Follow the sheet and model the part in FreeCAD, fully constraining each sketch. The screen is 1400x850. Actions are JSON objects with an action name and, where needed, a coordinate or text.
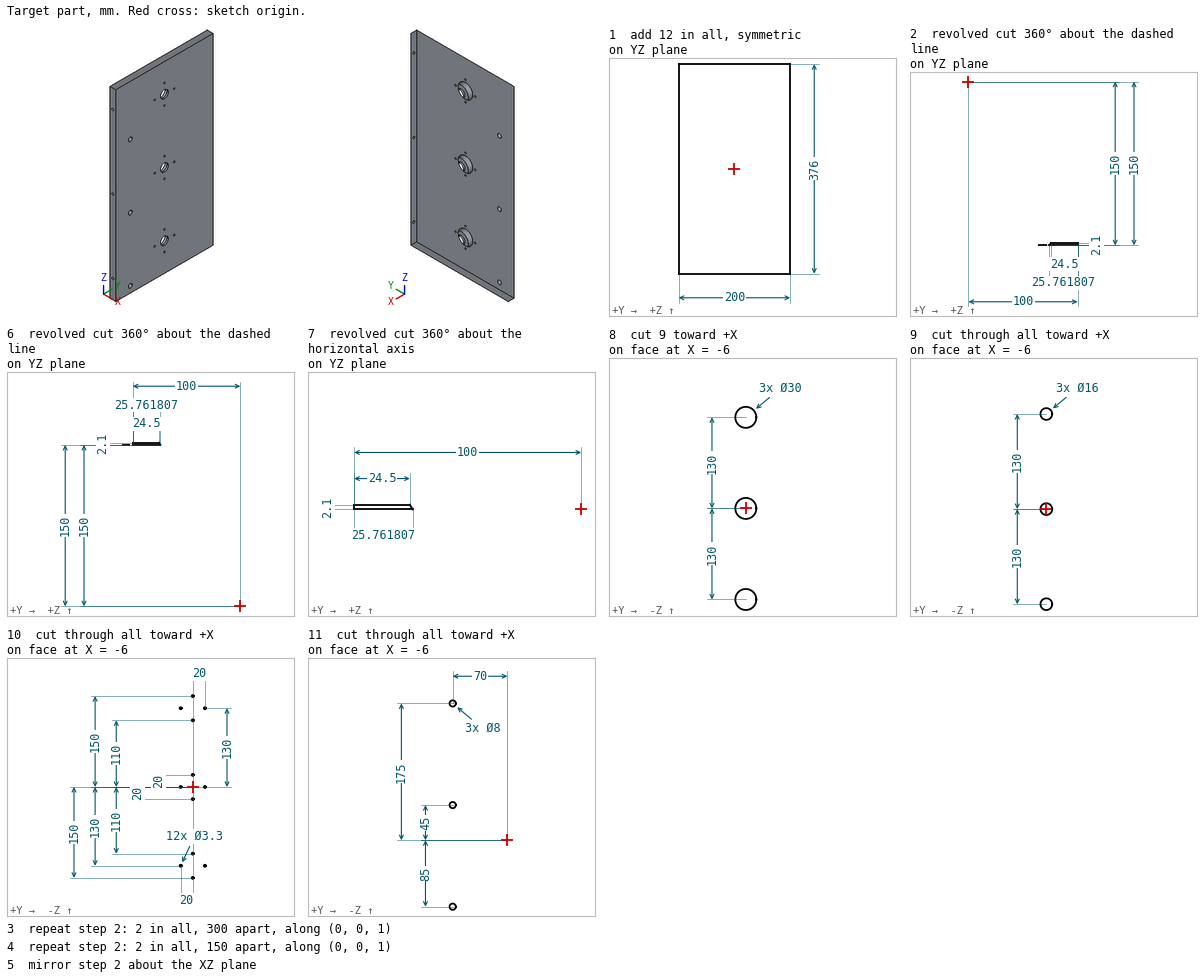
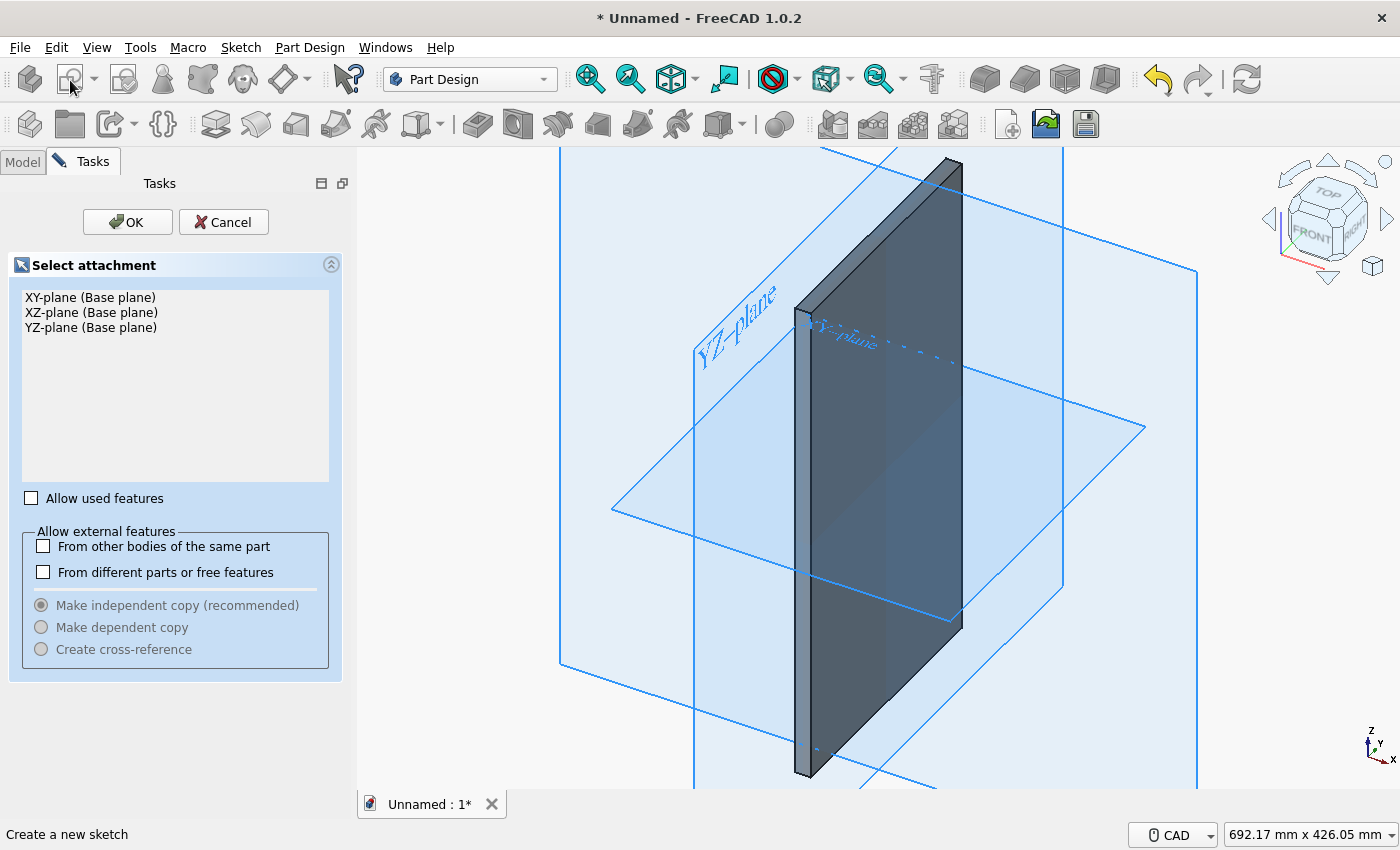
{"action": "left_click", "coordinate": [82, 328]}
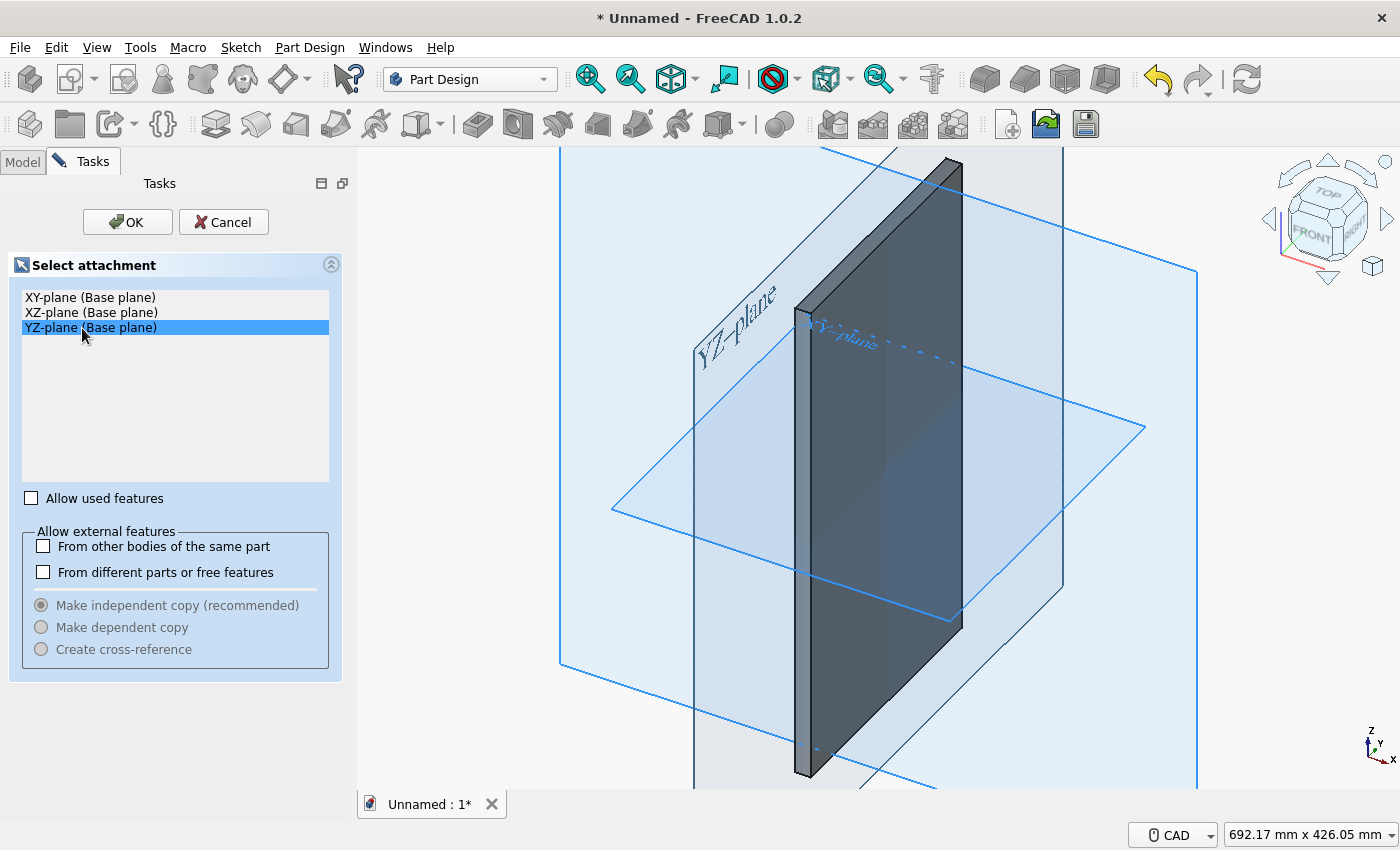
{"action": "left_click", "coordinate": [128, 222]}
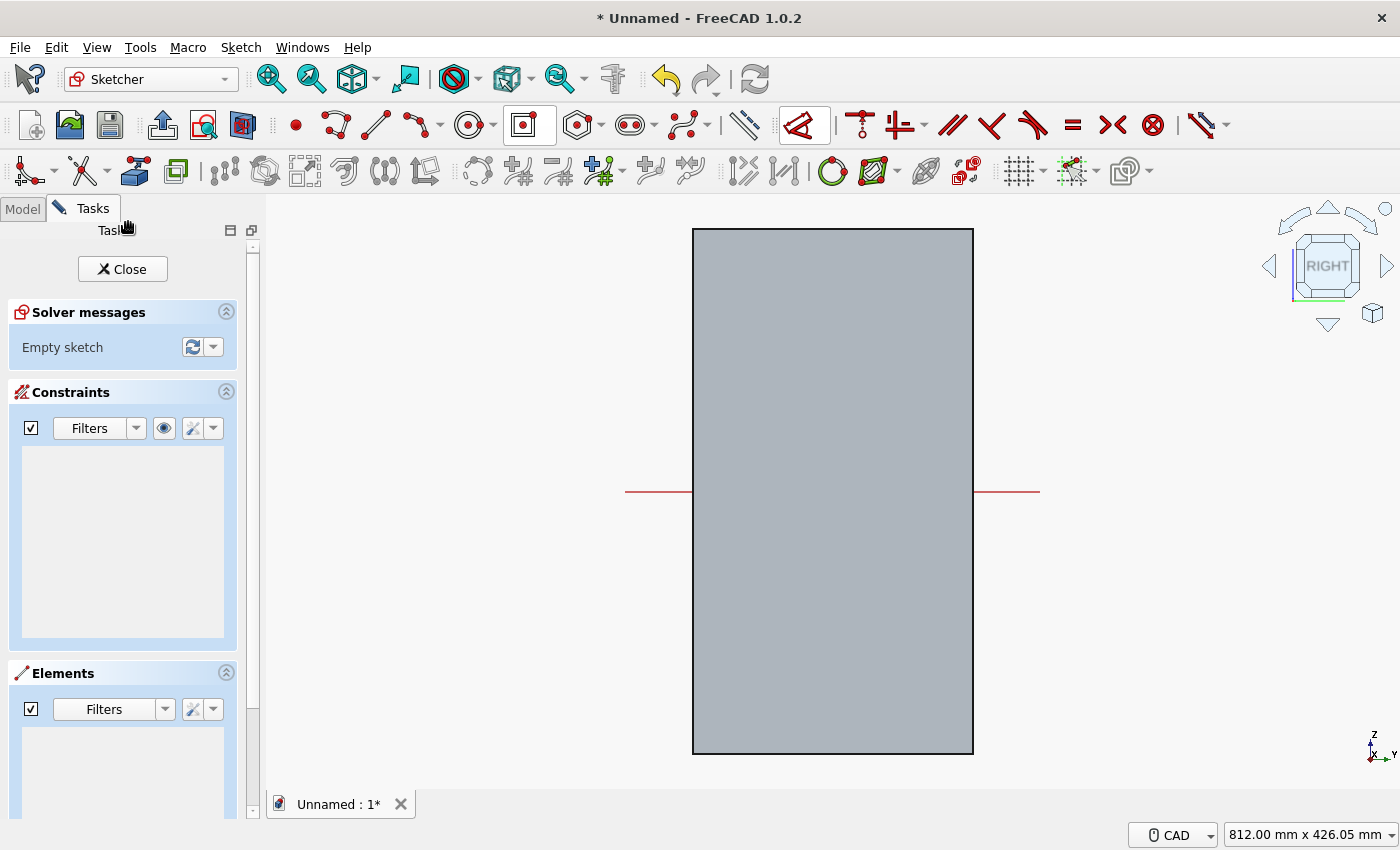
{"action": "left_click", "coordinate": [244, 126]}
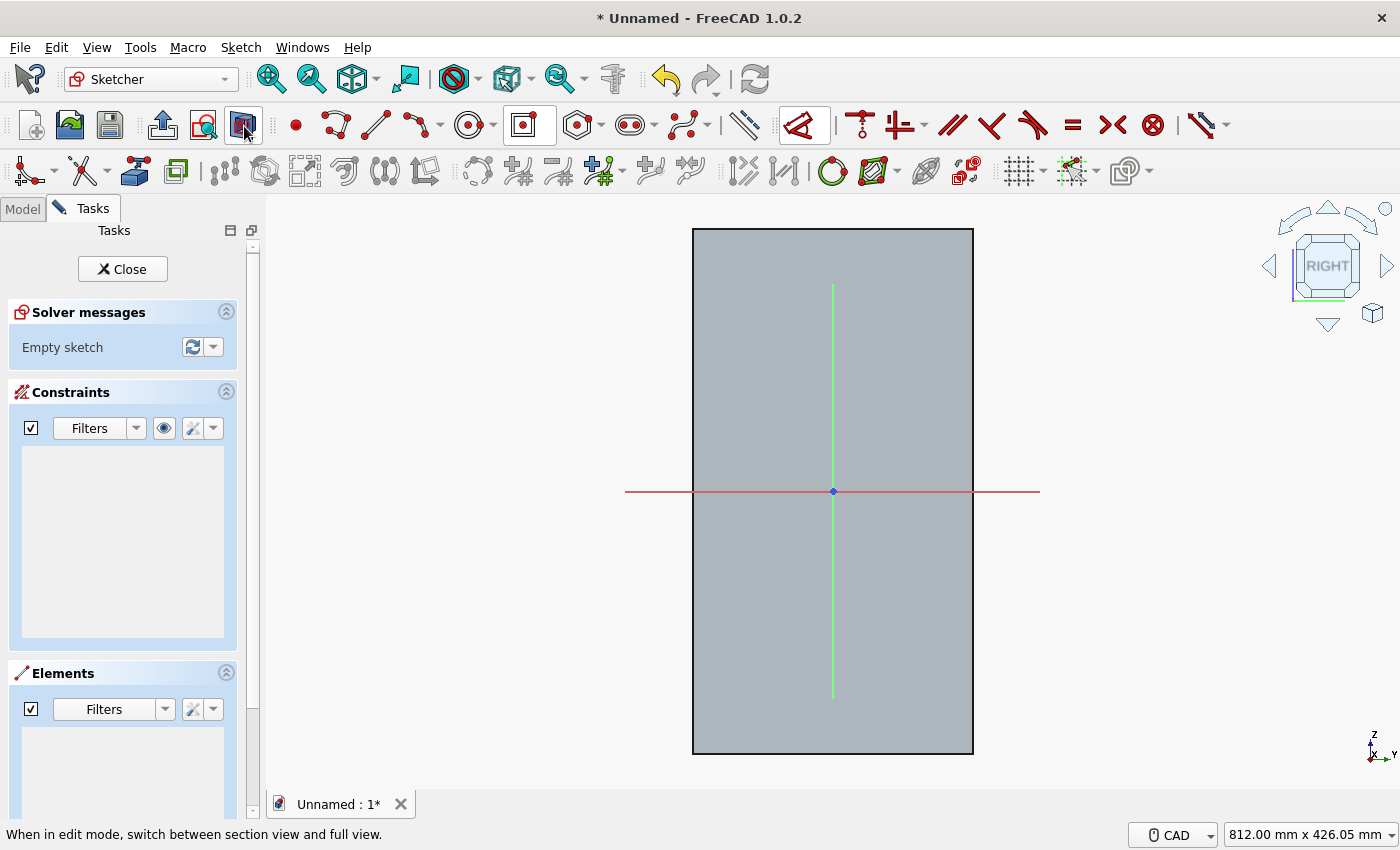
{"action": "scroll", "coordinate": [962, 716], "scroll_direction": "up", "scroll_amount": 13}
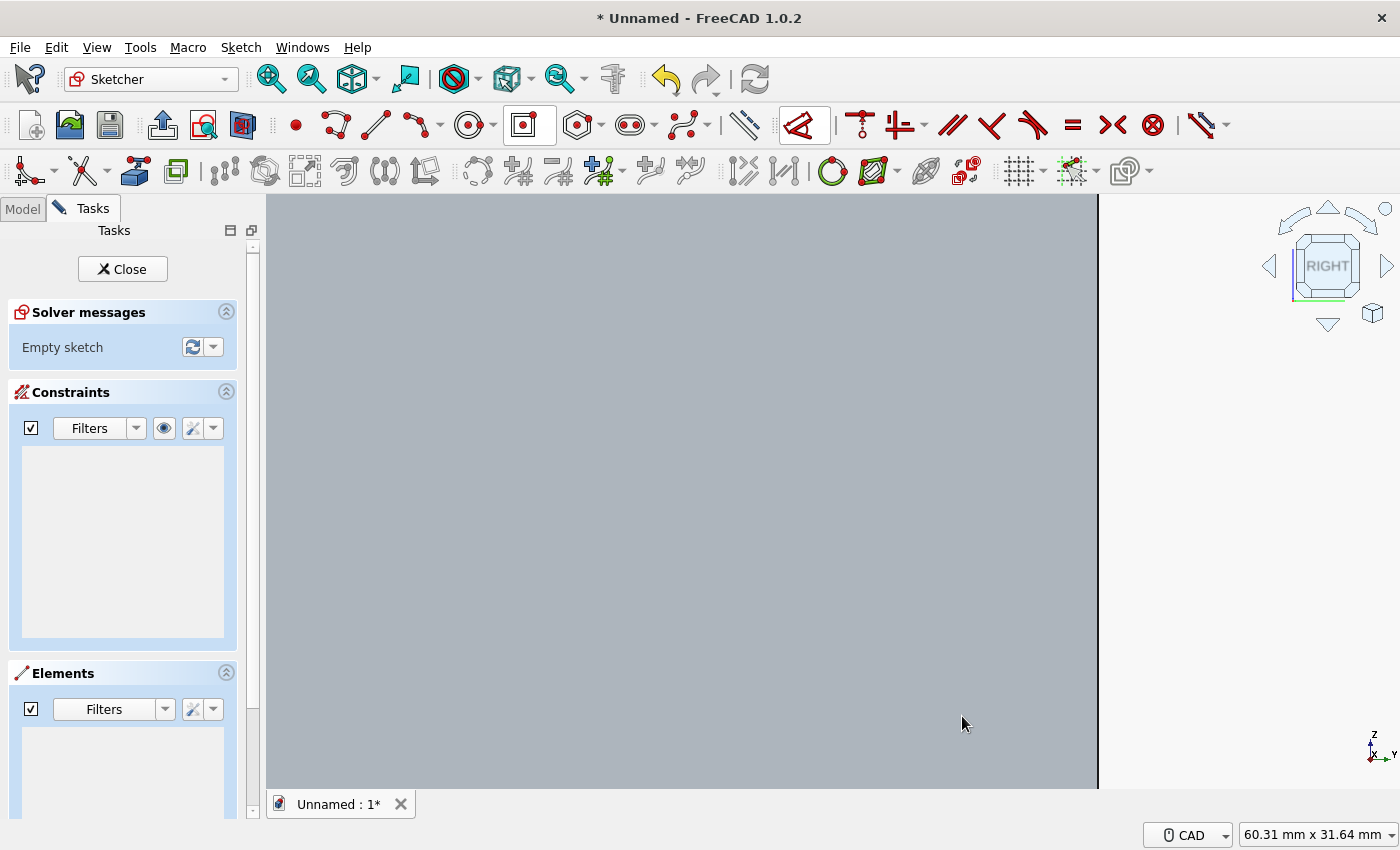
{"action": "left_click", "coordinate": [336, 126]}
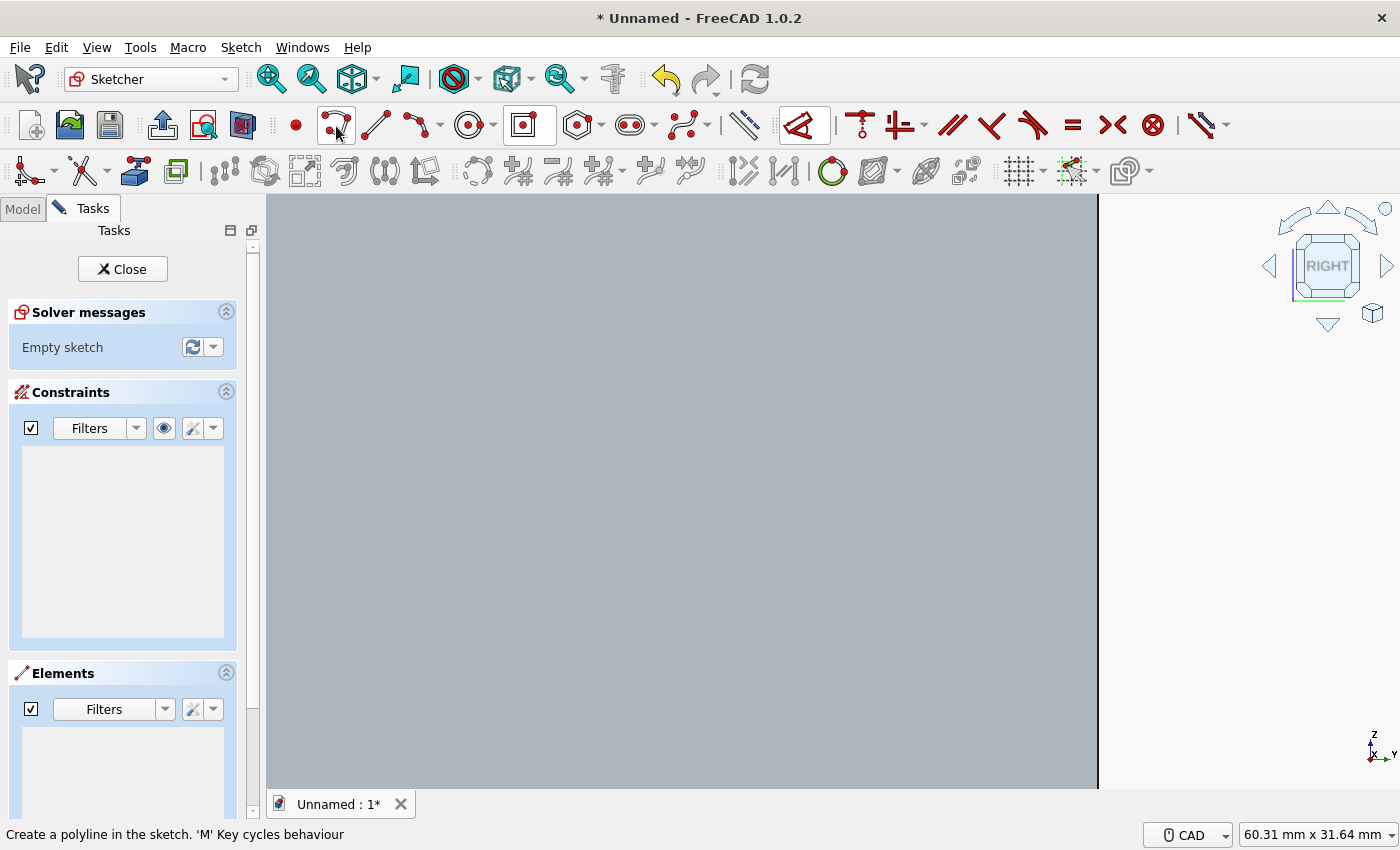
{"action": "left_click", "coordinate": [637, 463]}
{"action": "left_click", "coordinate": [613, 503]}
{"action": "left_click", "coordinate": [1098, 503]}
{"action": "left_click", "coordinate": [1098, 463]}
{"action": "left_click", "coordinate": [637, 464]}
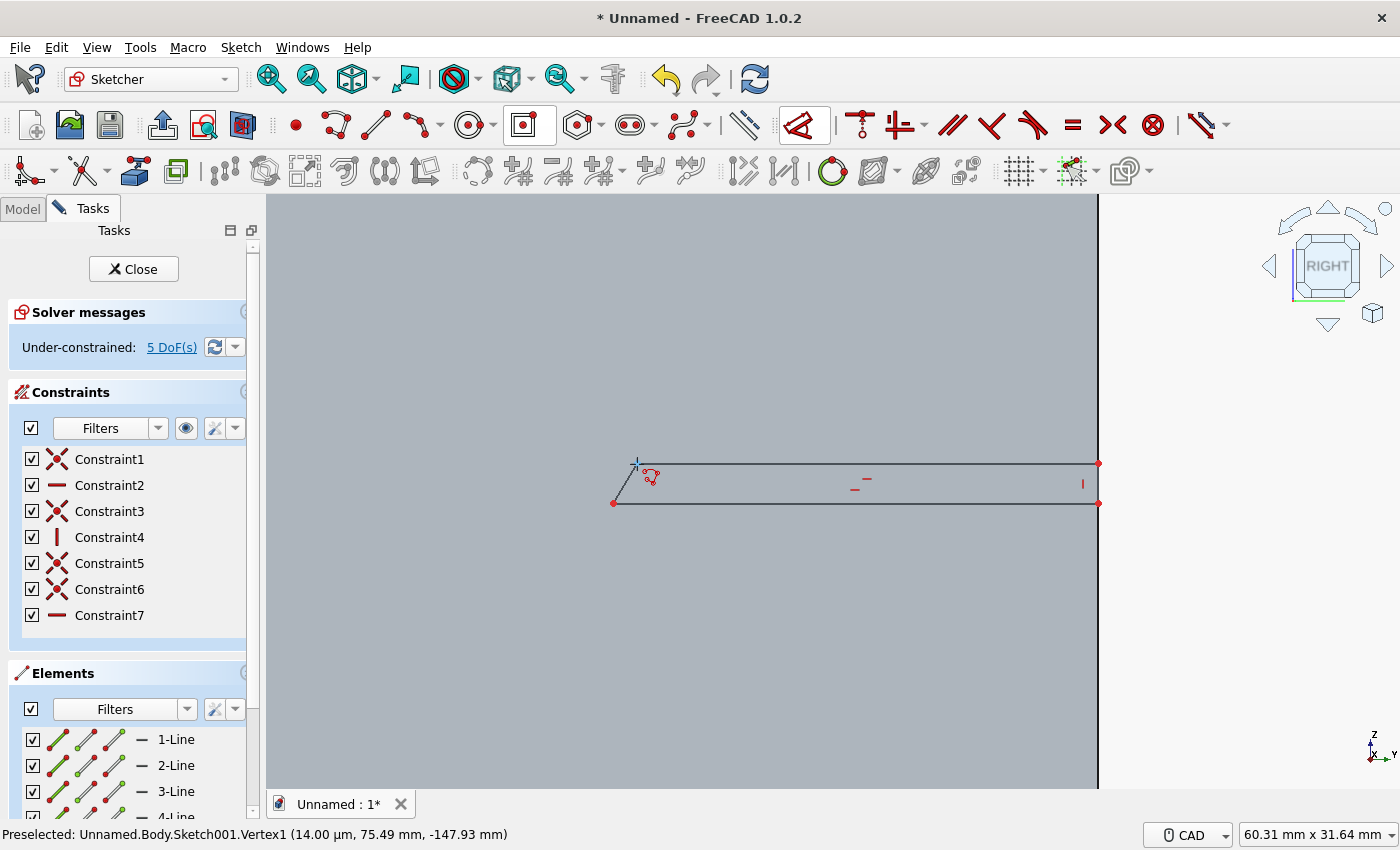
{"action": "left_click", "coordinate": [376, 126]}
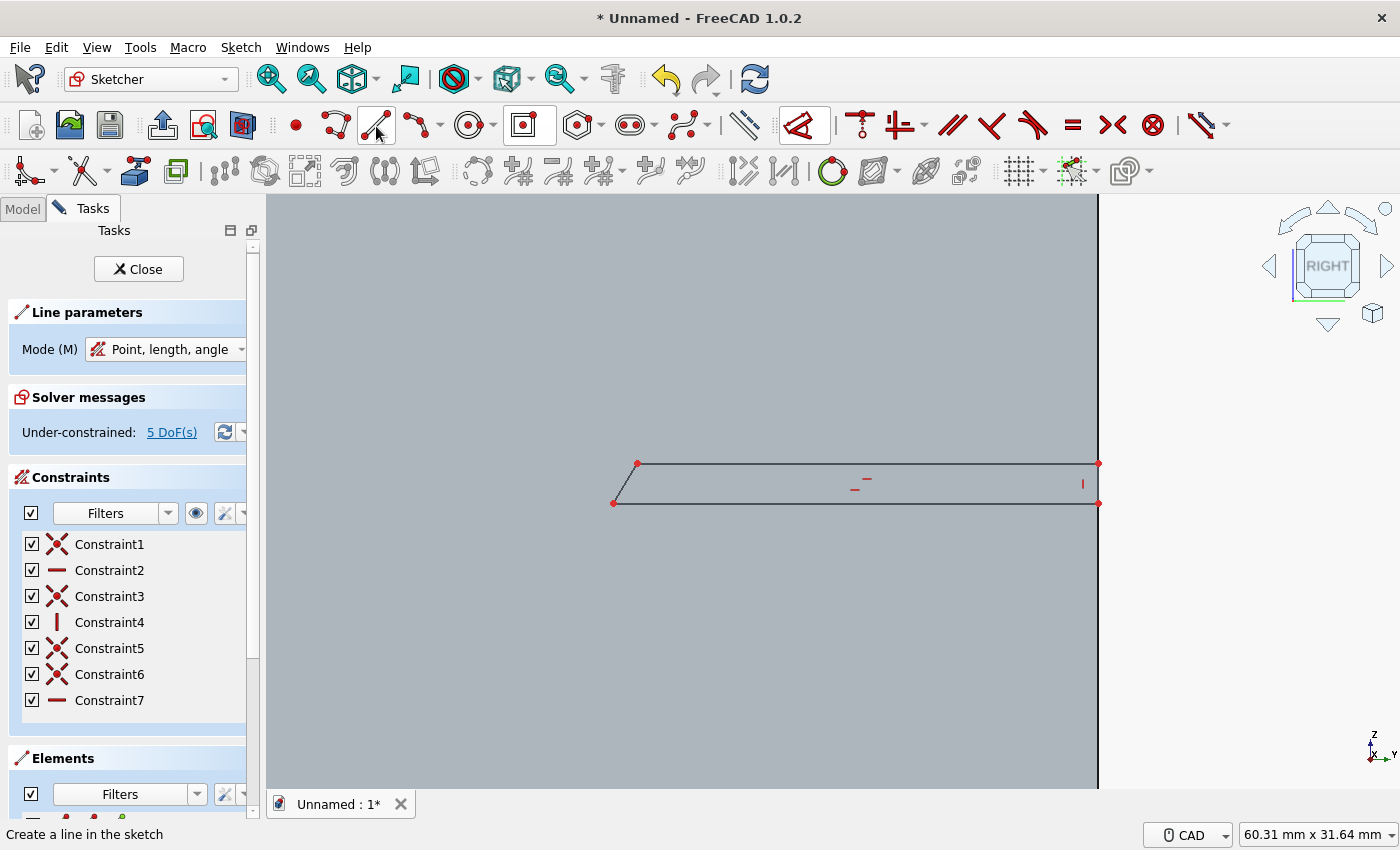
{"action": "left_click", "coordinate": [565, 503]}
{"action": "left_click", "coordinate": [420, 503]}
{"action": "key", "text": "Escape"}